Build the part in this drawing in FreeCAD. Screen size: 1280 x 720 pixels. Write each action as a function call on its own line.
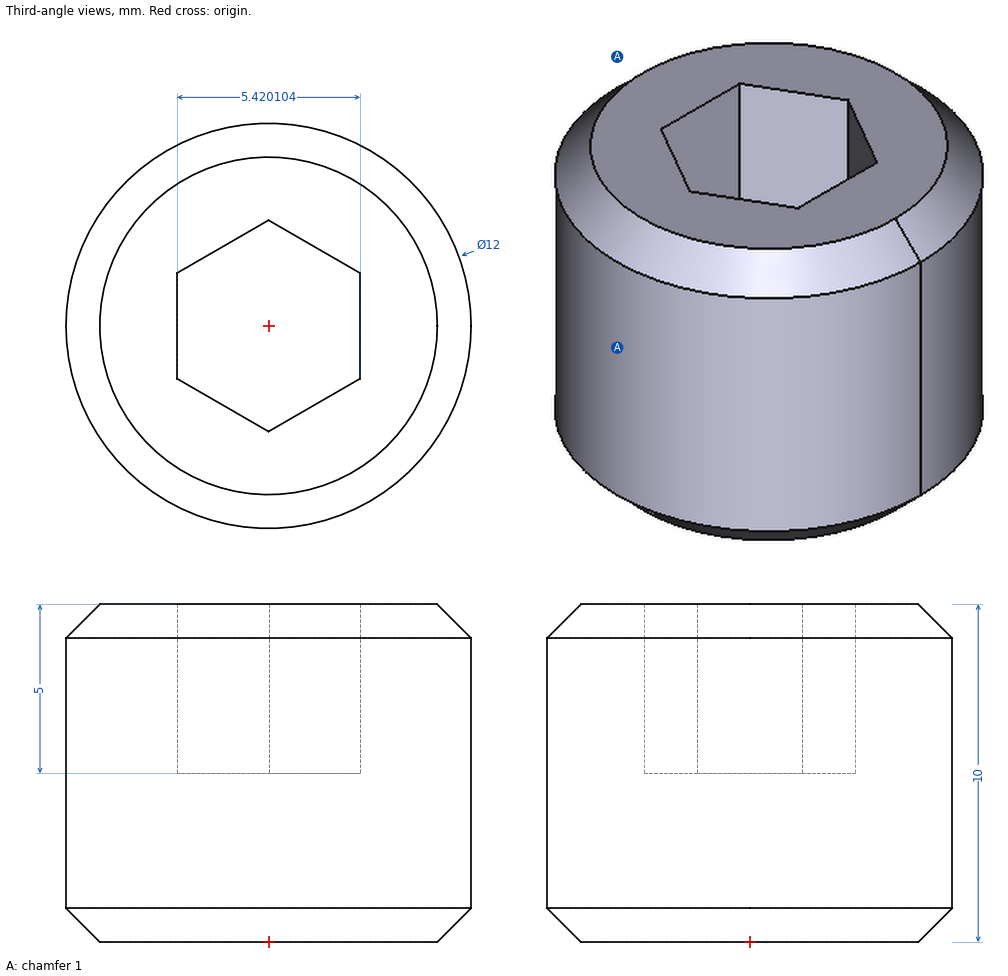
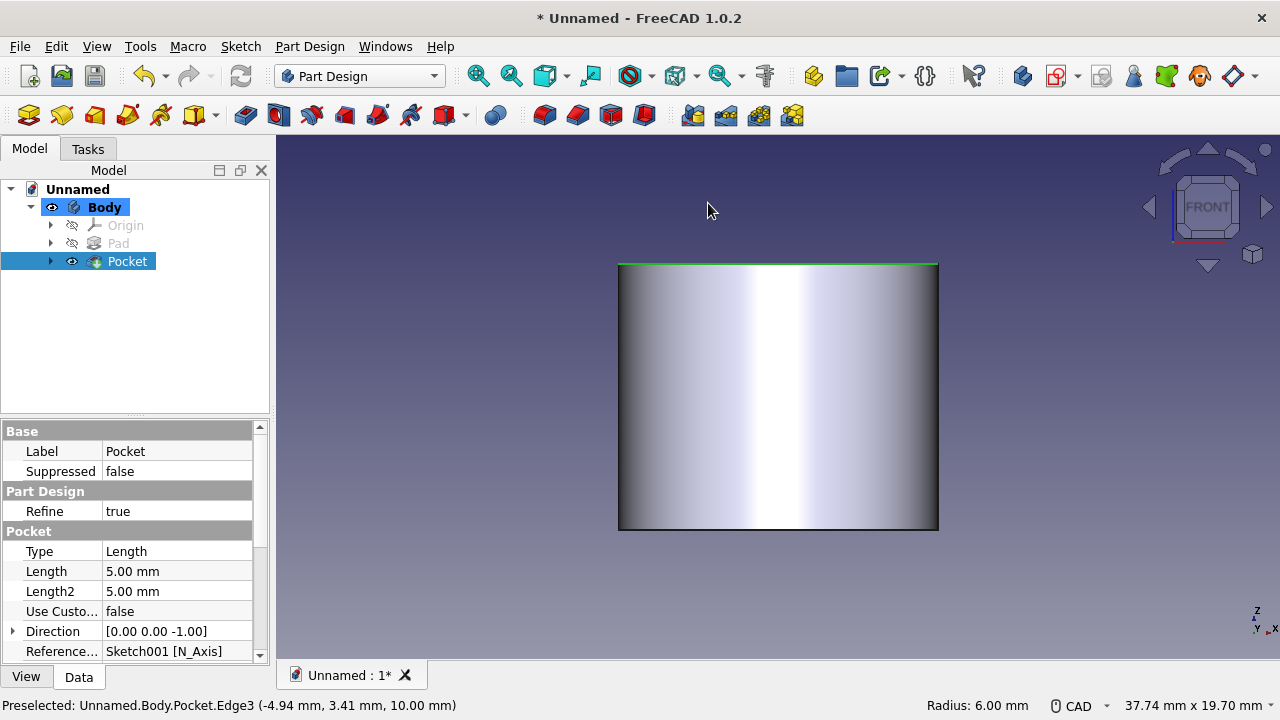
click(649, 529, ctrl)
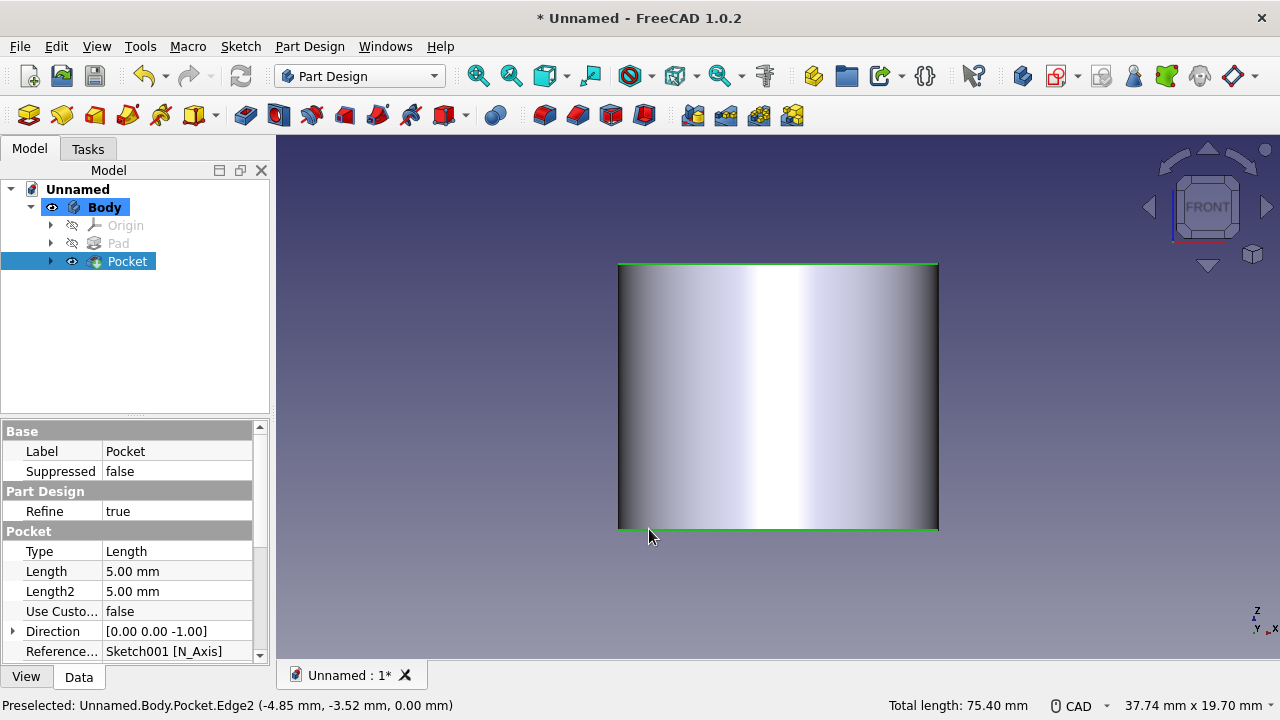
click(578, 116)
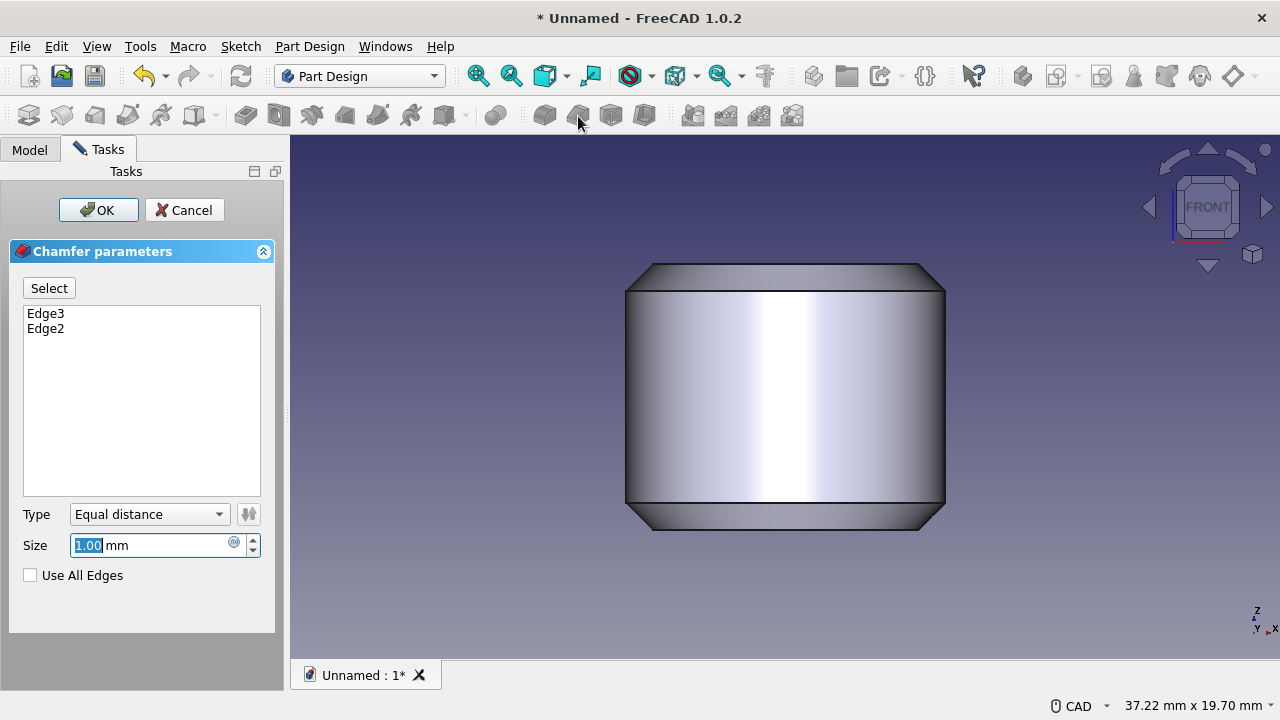
text(1)
key(Tab)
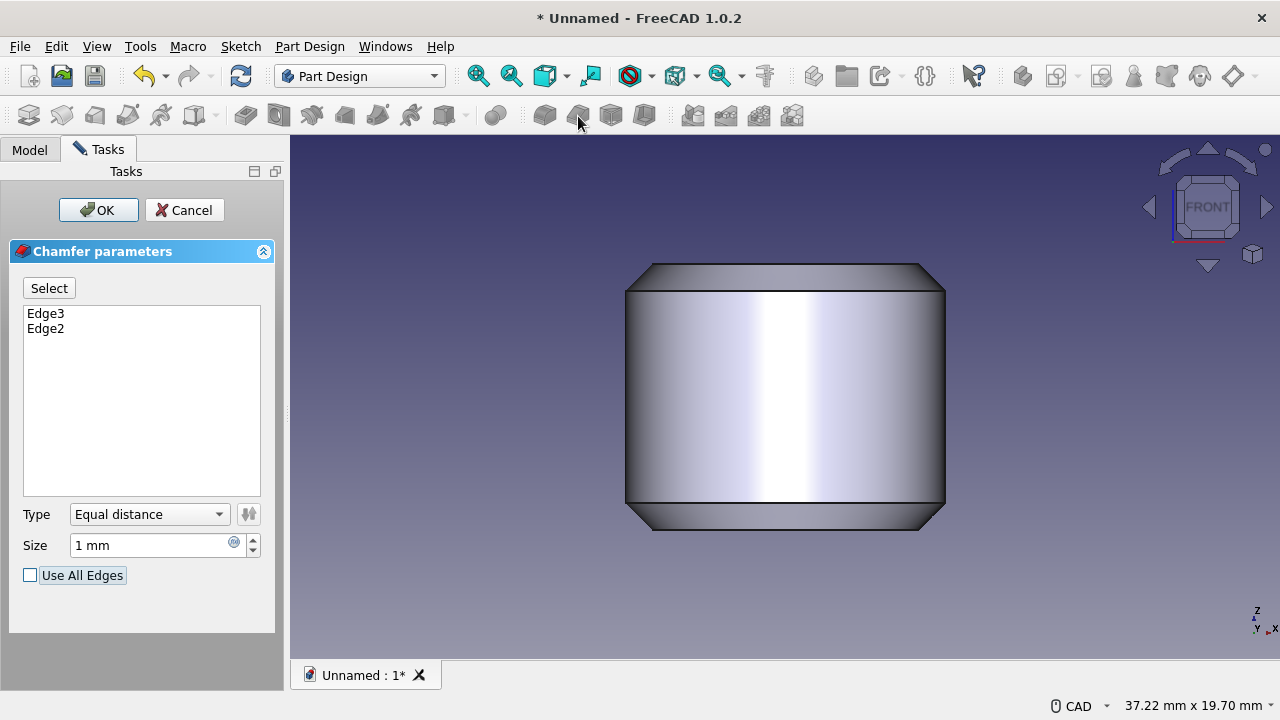
click(99, 210)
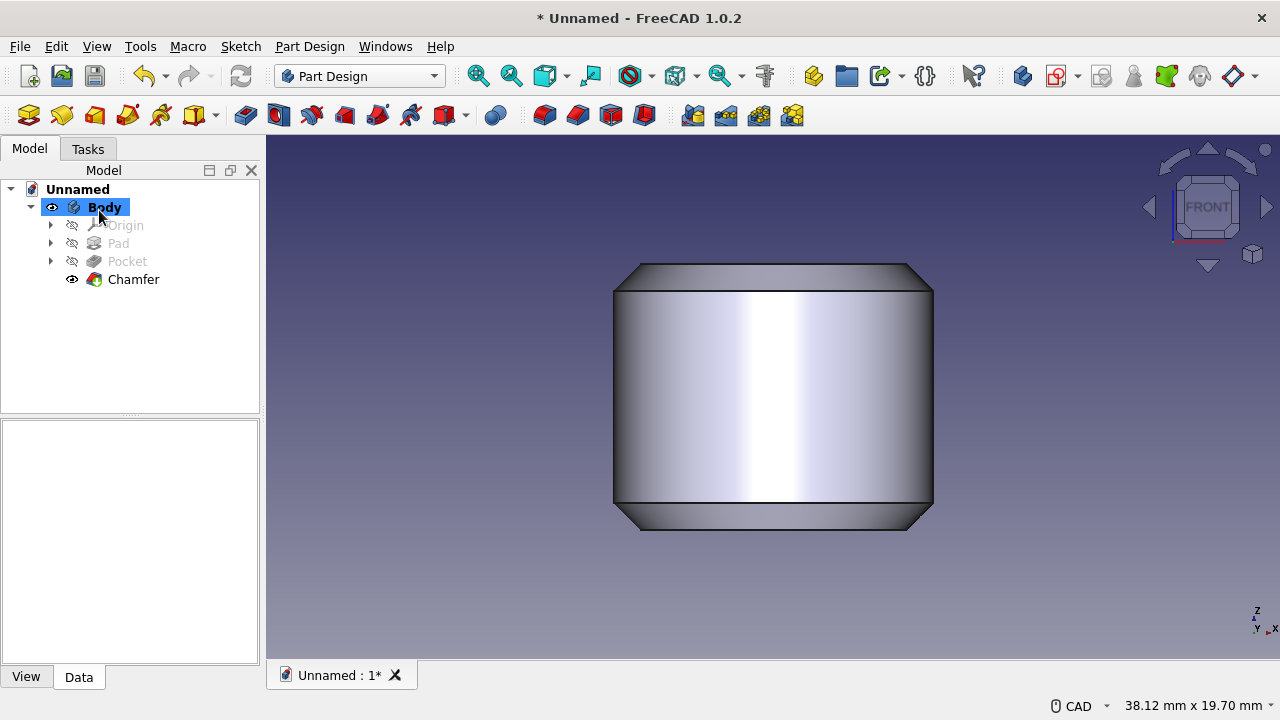
key(0)